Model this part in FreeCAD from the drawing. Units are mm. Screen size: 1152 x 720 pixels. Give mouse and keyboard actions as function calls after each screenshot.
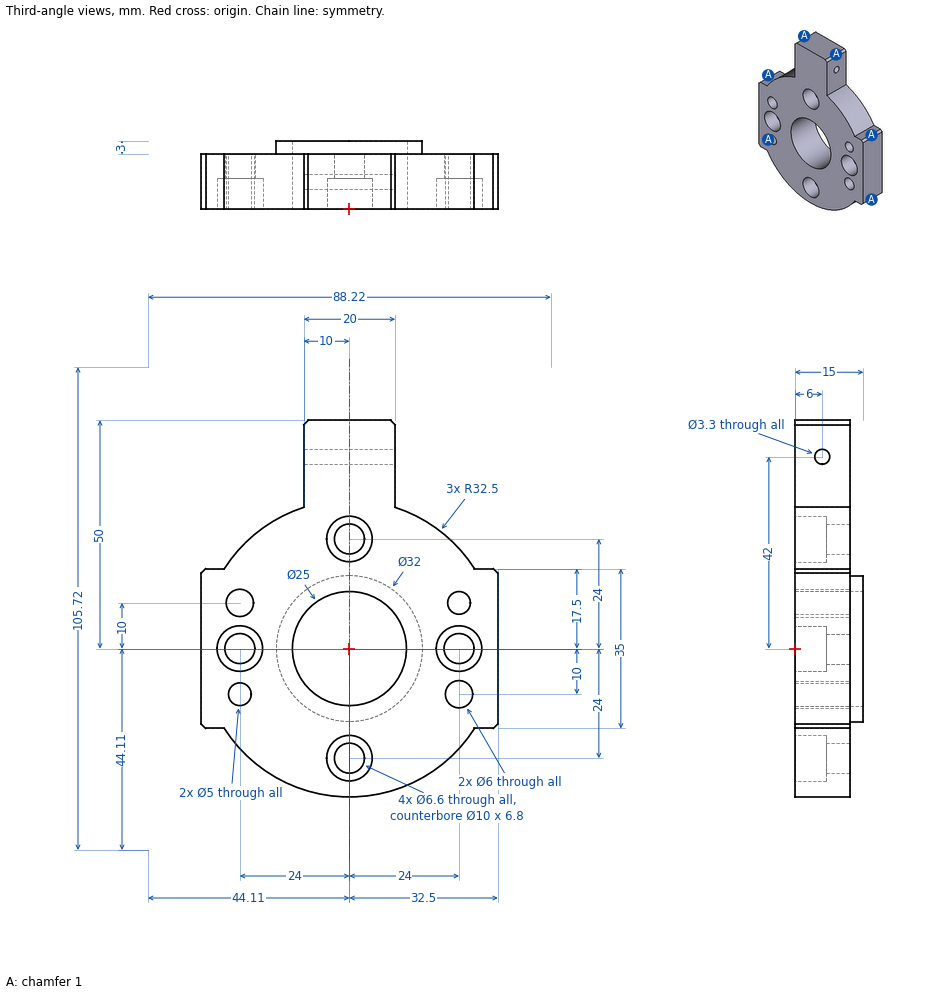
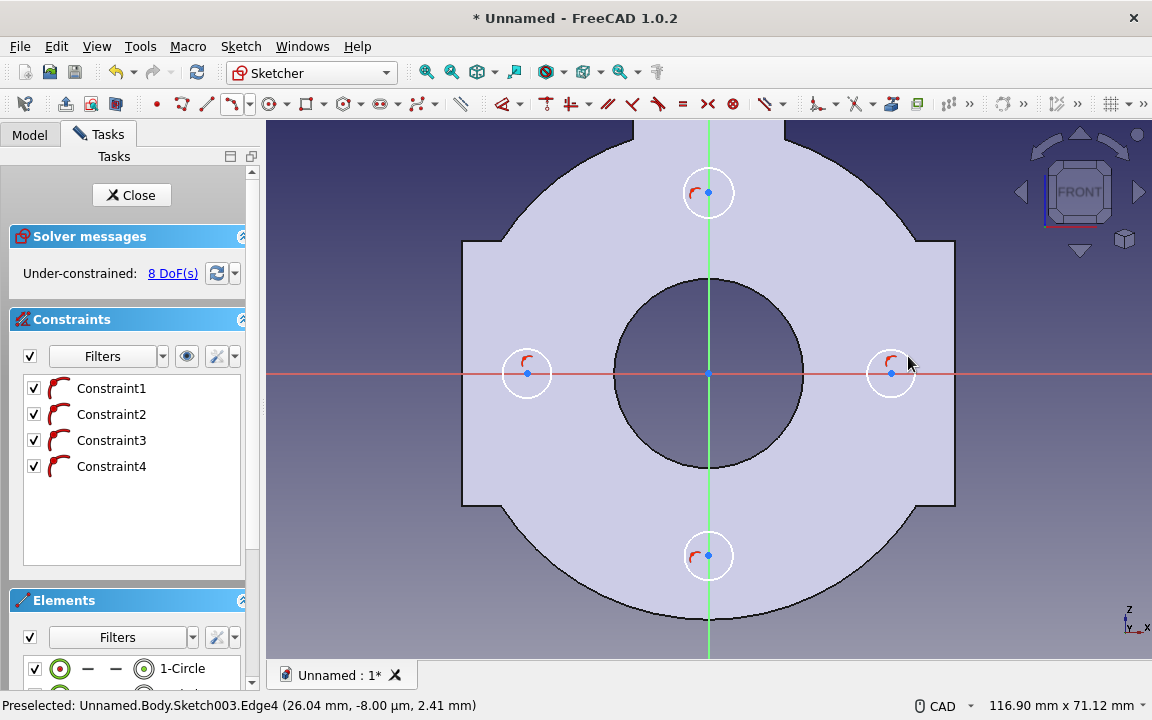
click(726, 539)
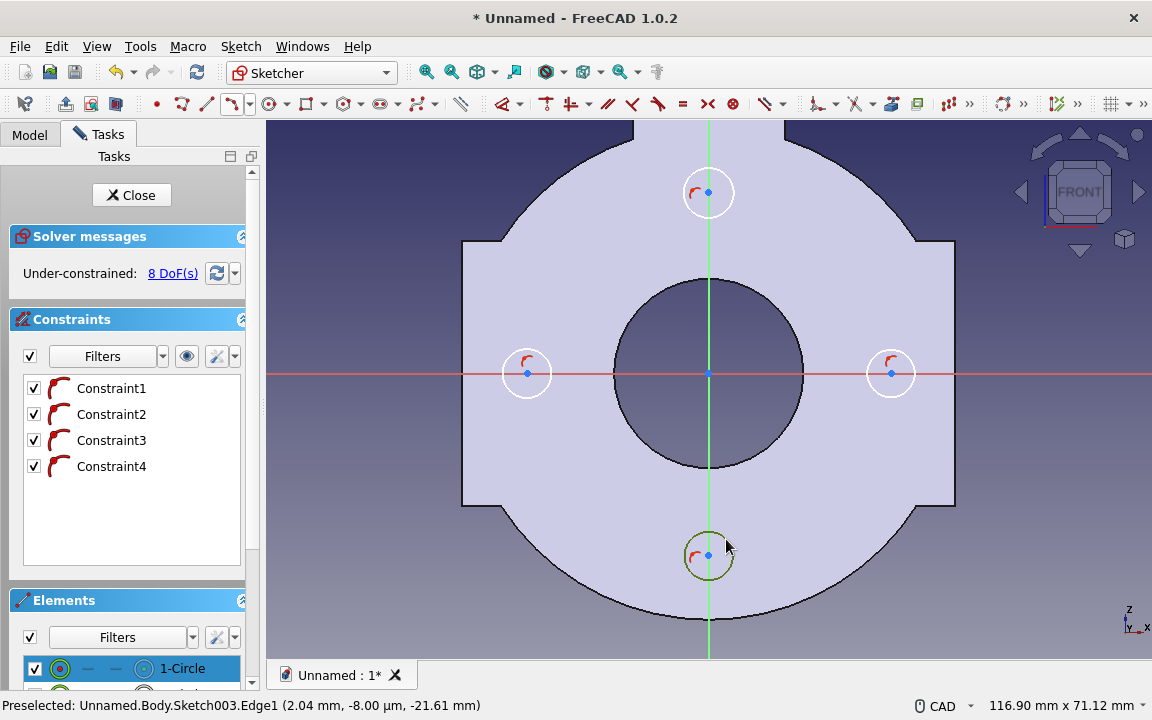
click(544, 356)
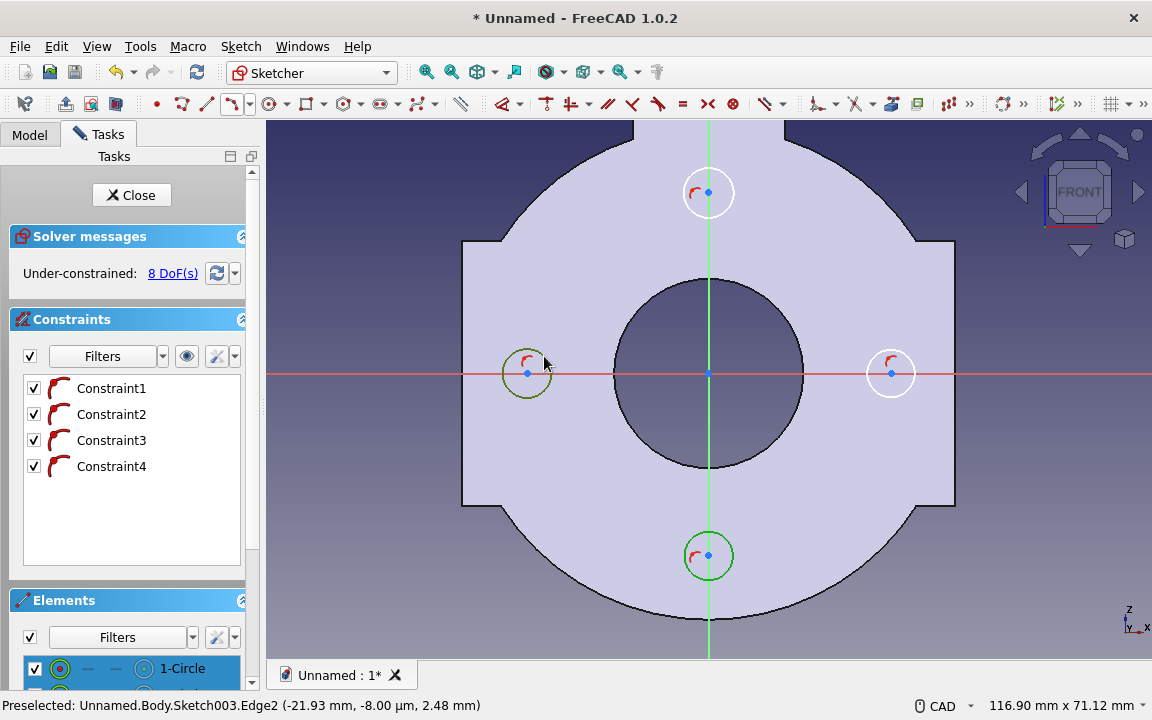
click(726, 175)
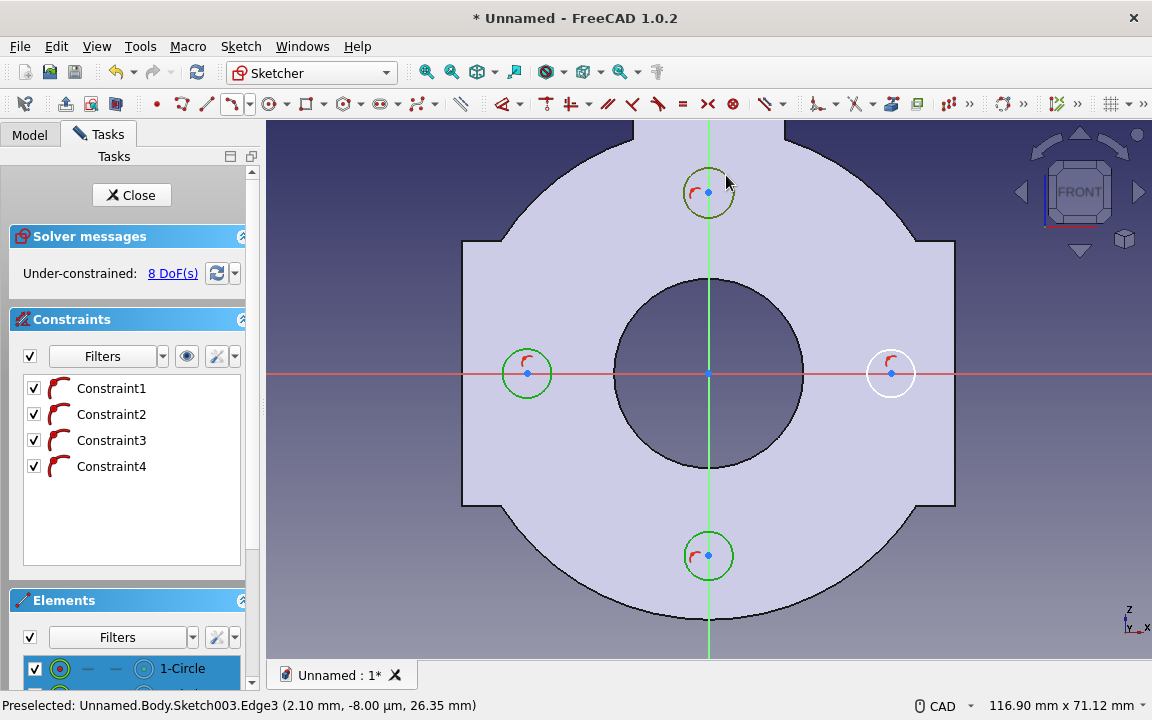
click(908, 357)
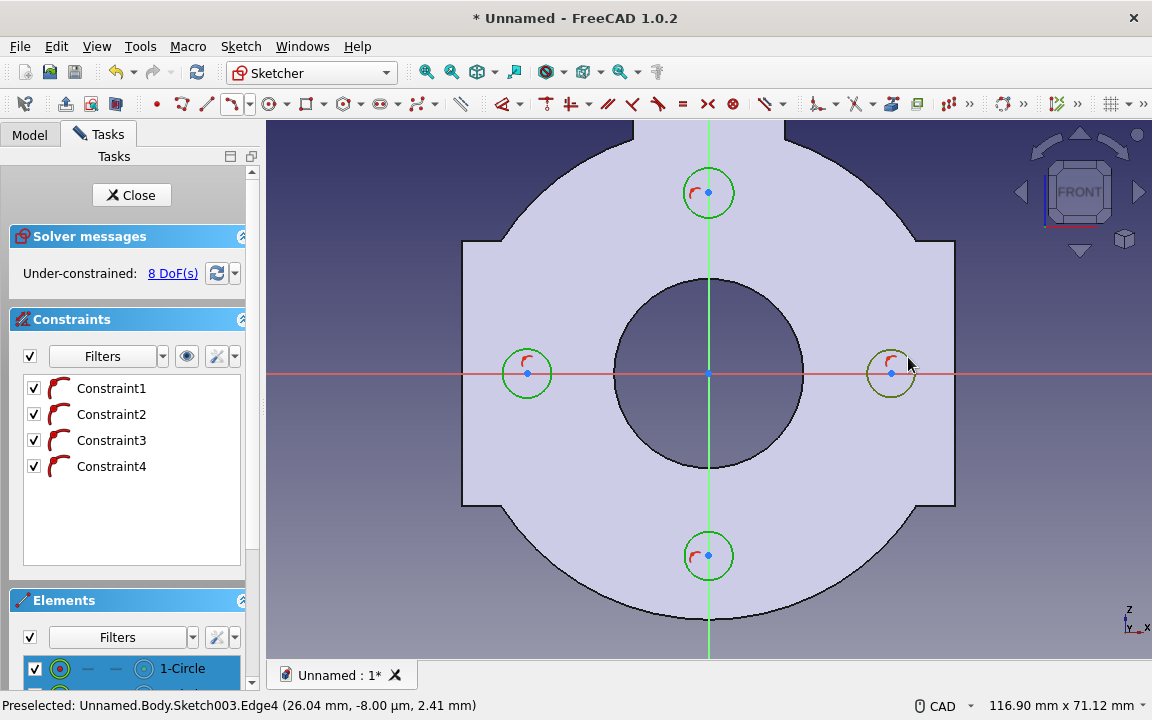
click(683, 104)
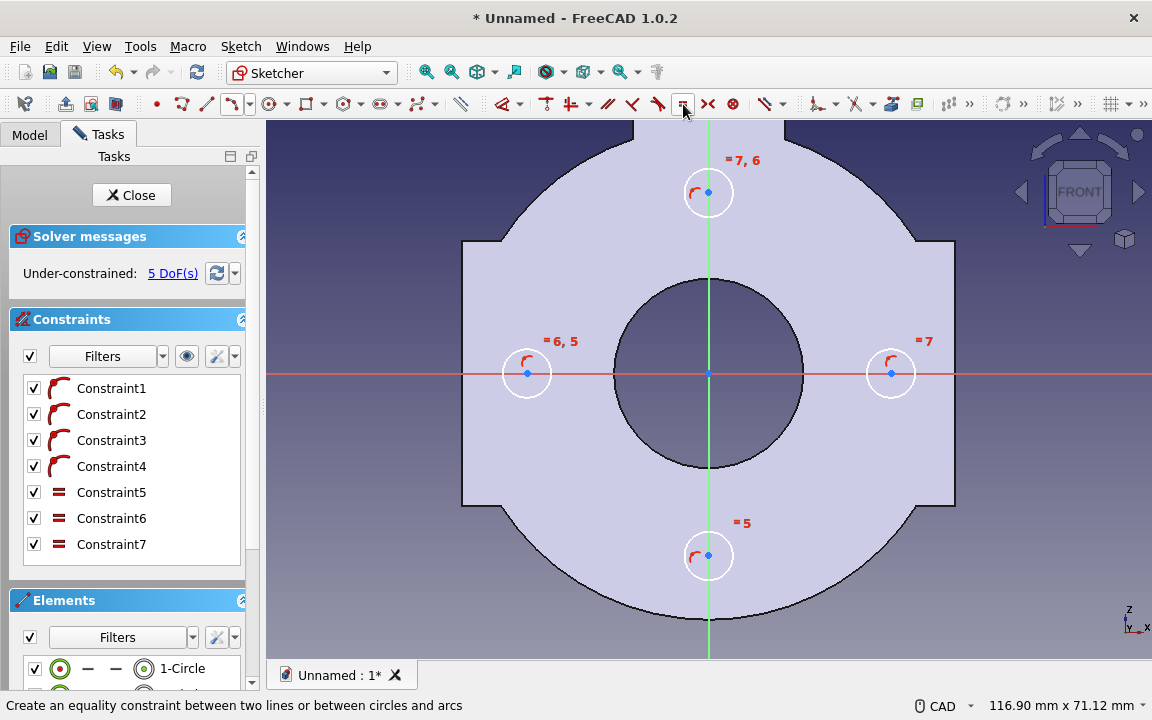
click(502, 104)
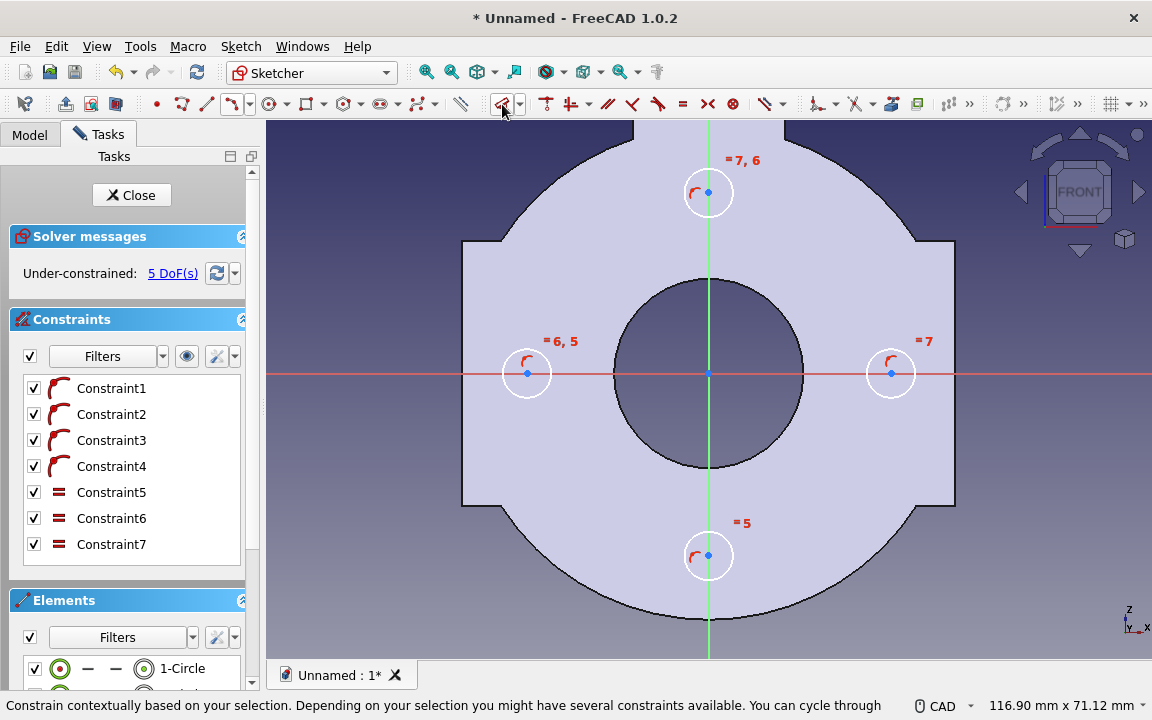
click(726, 539)
click(749, 517)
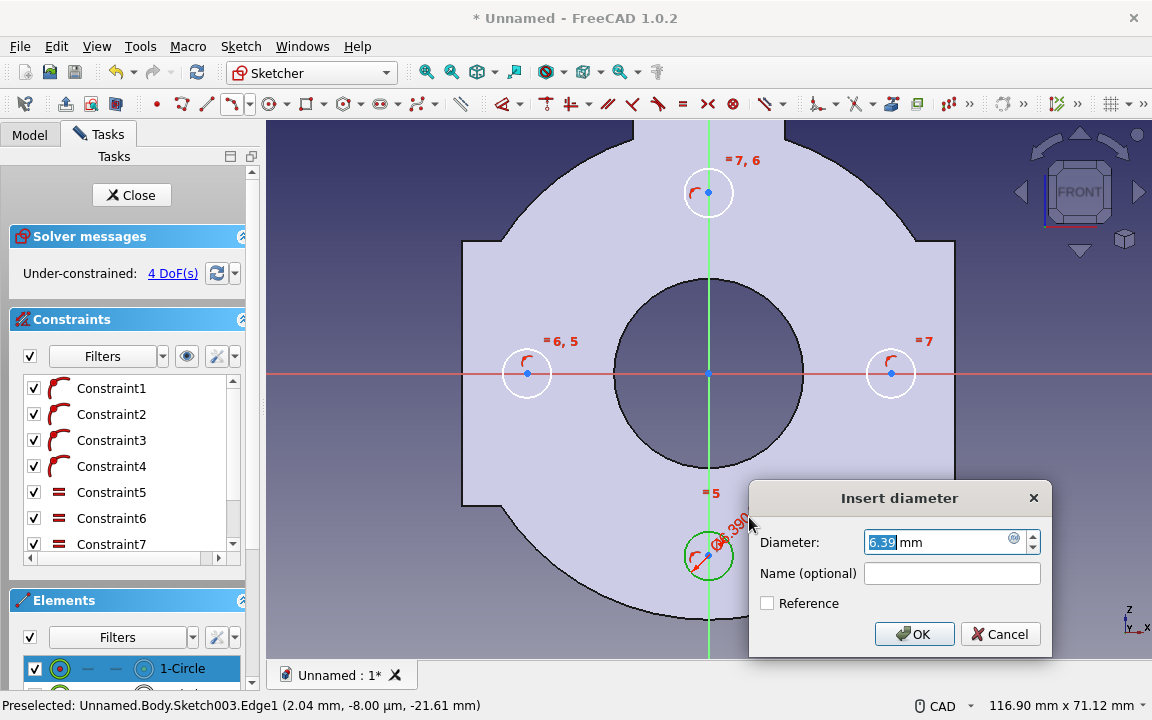
text(6.6)
key(Return)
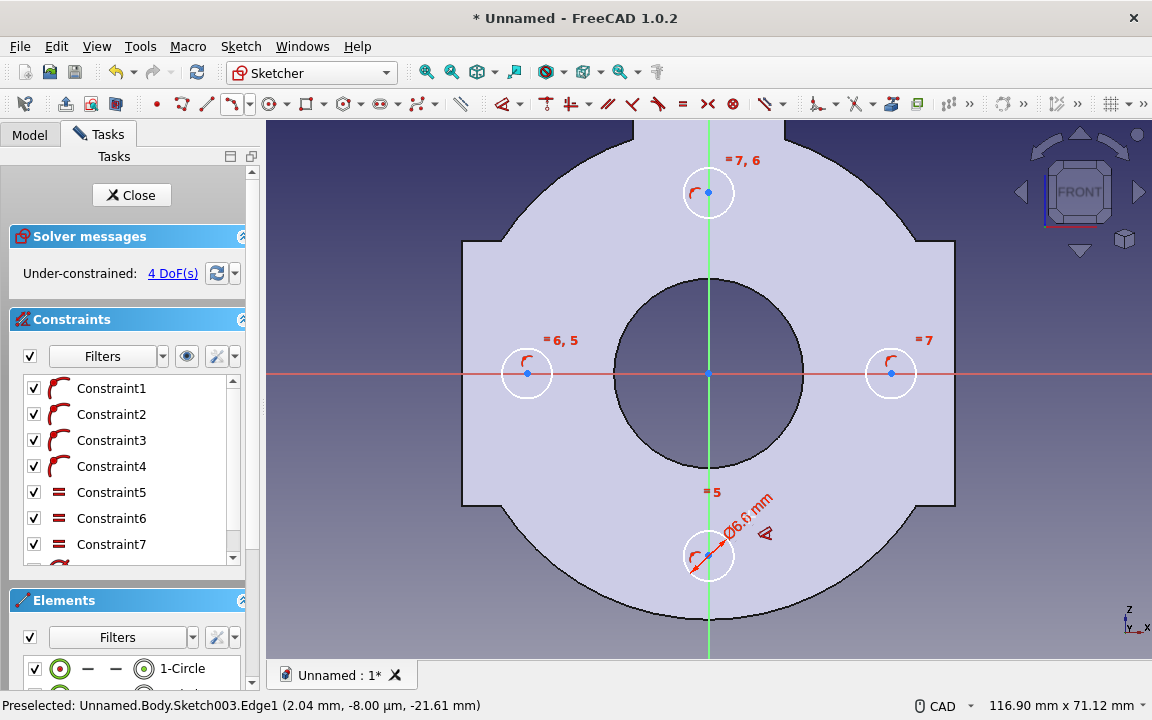
click(709, 556)
click(743, 465)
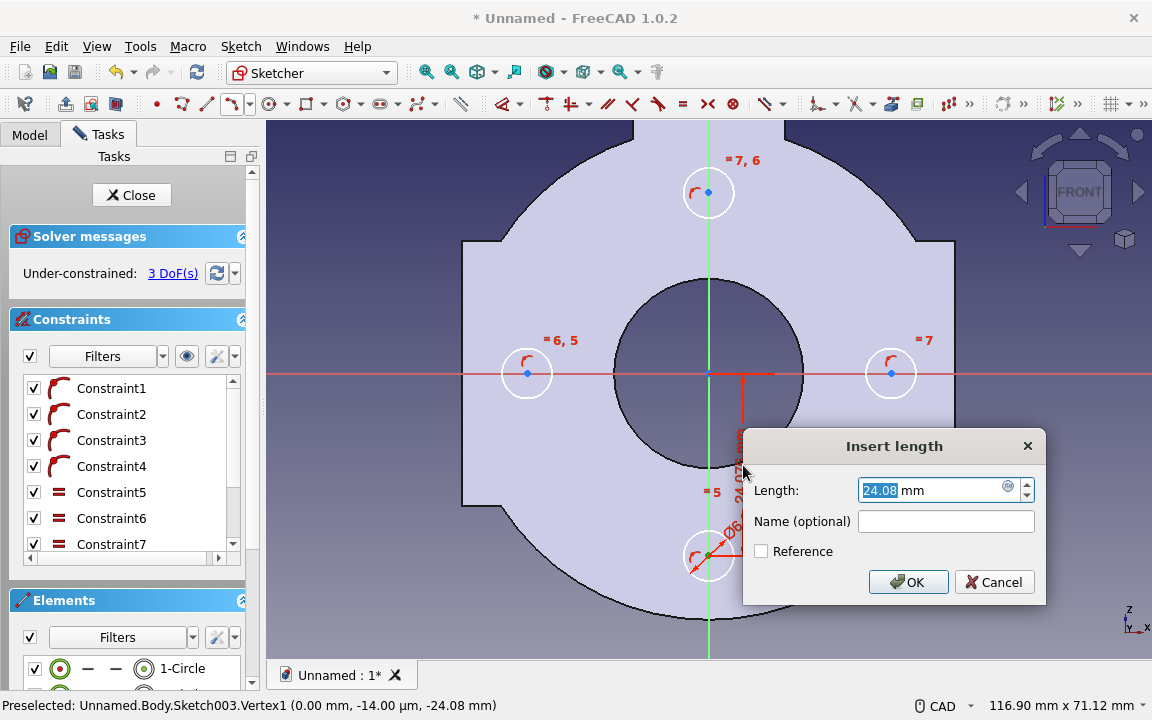
text(24)
key(Return)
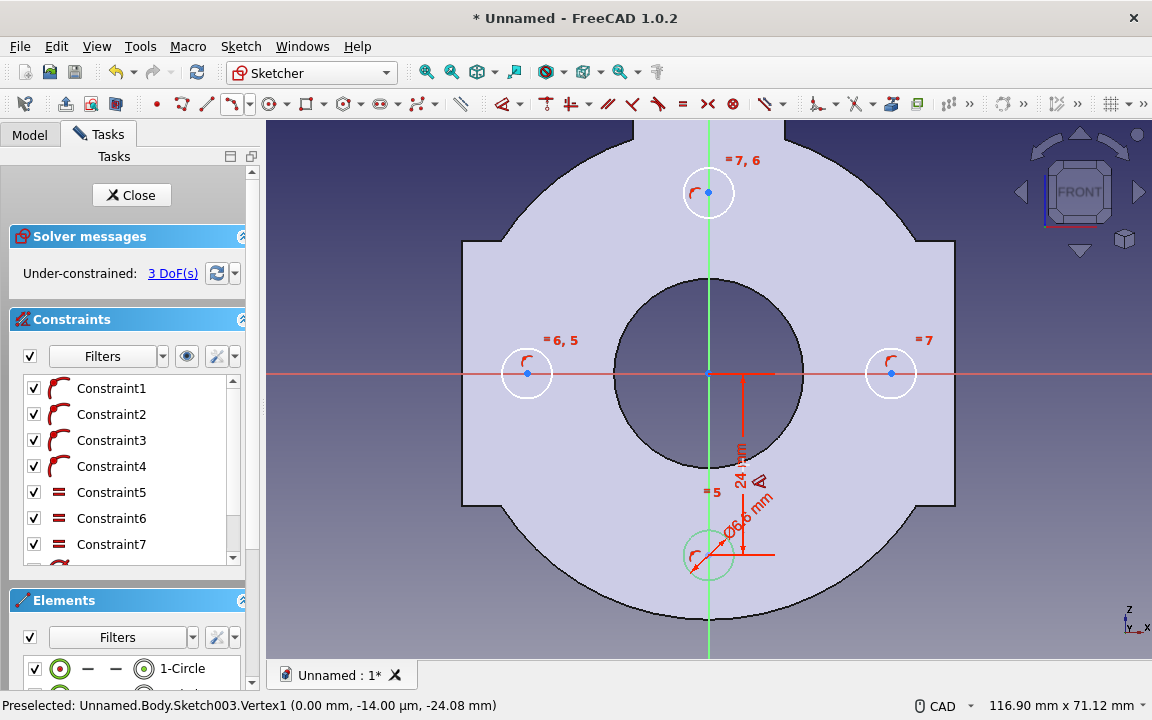
click(527, 374)
click(618, 408)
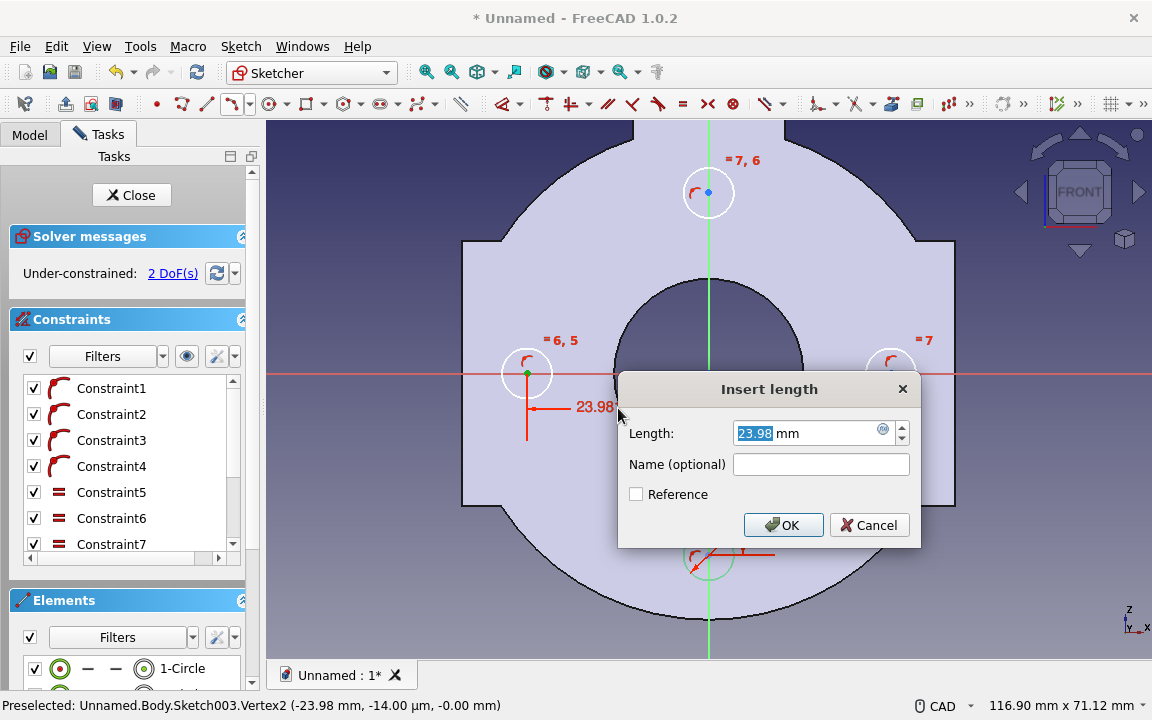
text(24)
key(Return)